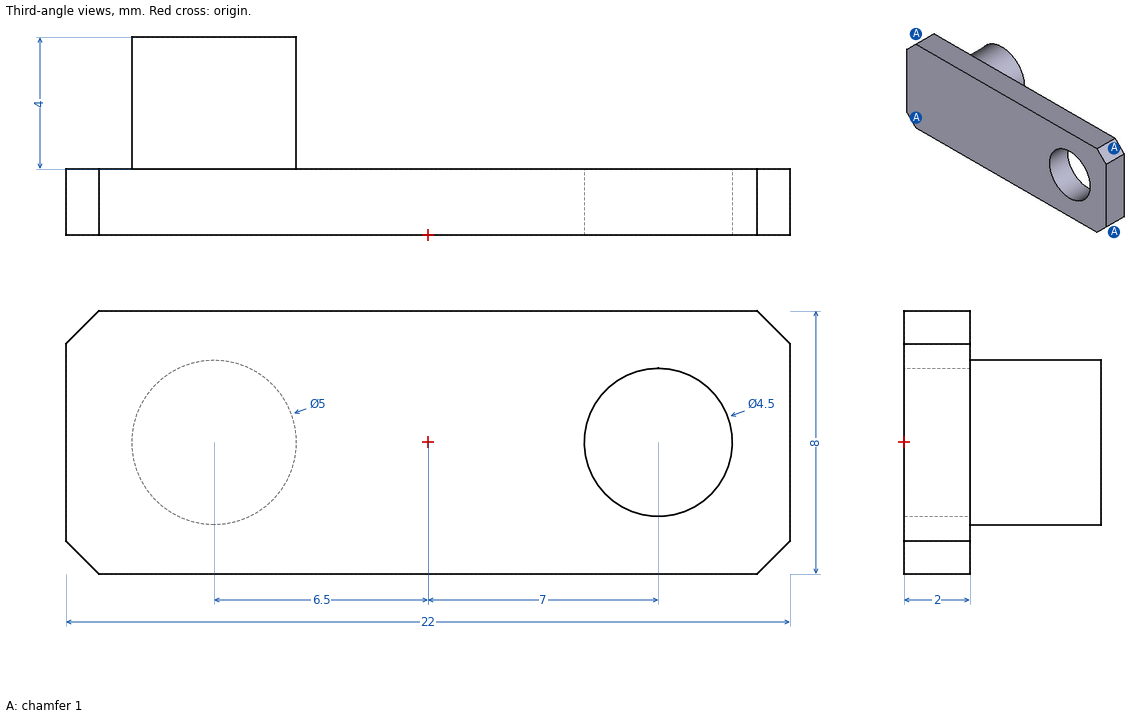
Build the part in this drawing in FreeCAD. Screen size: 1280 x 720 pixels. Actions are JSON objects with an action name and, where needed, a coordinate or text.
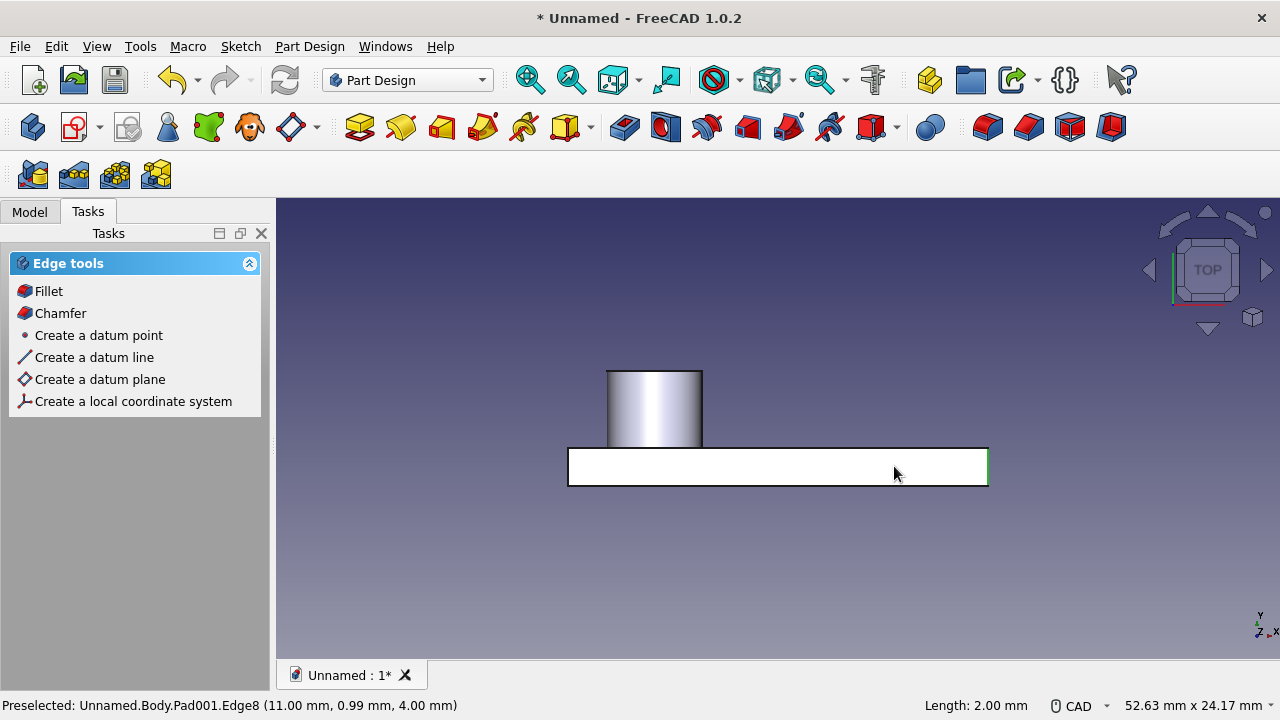
{"action": "left_click", "coordinate": [531, 80]}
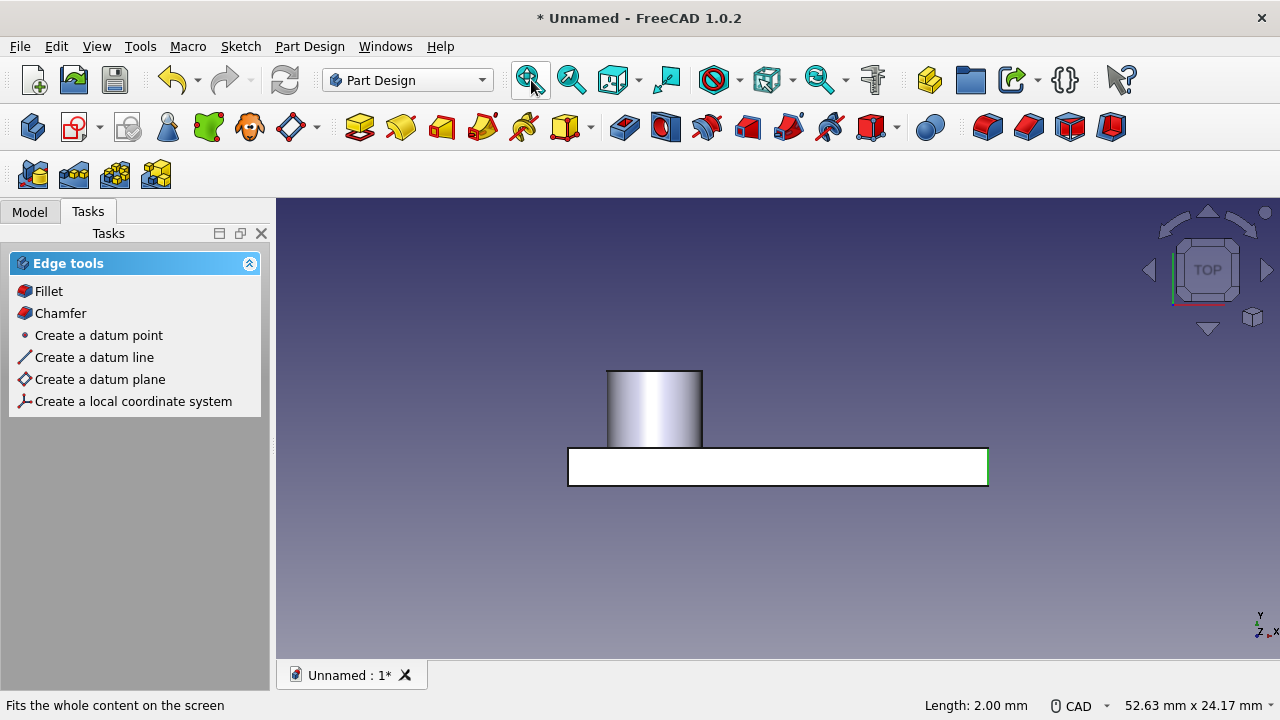
{"action": "left_click", "coordinate": [568, 466], "text": "ctrl"}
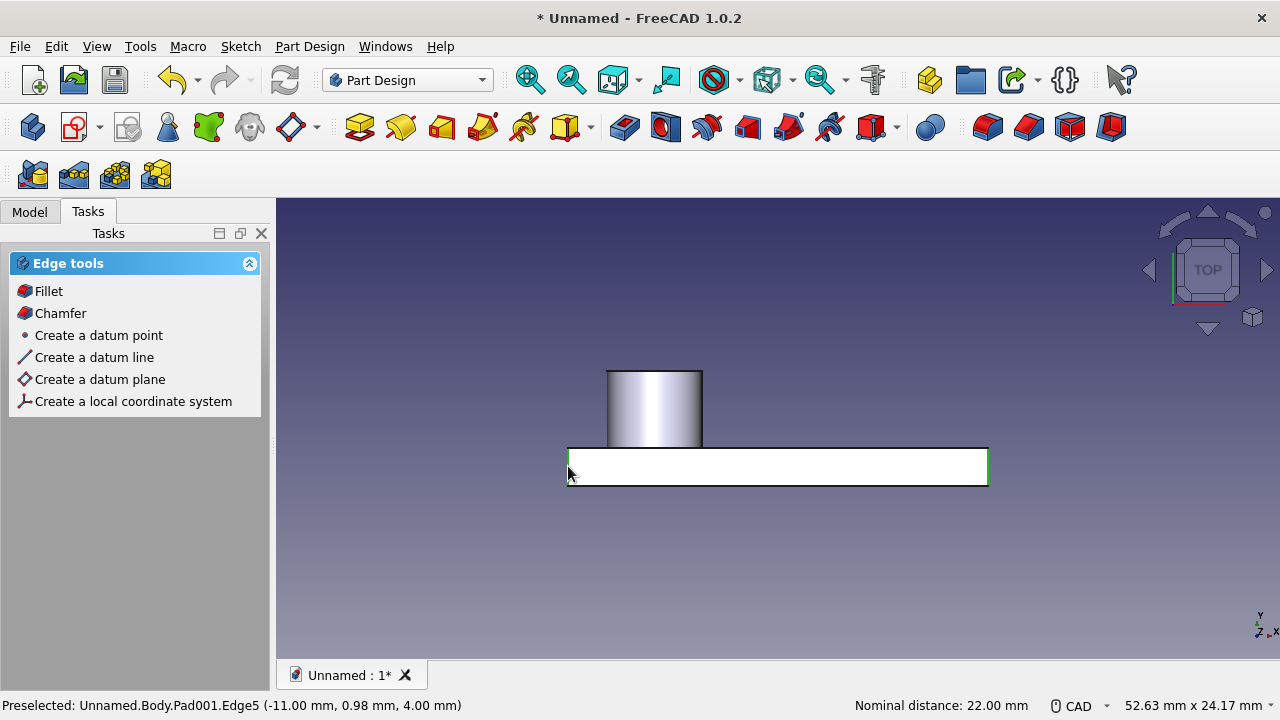
{"action": "key", "text": "1"}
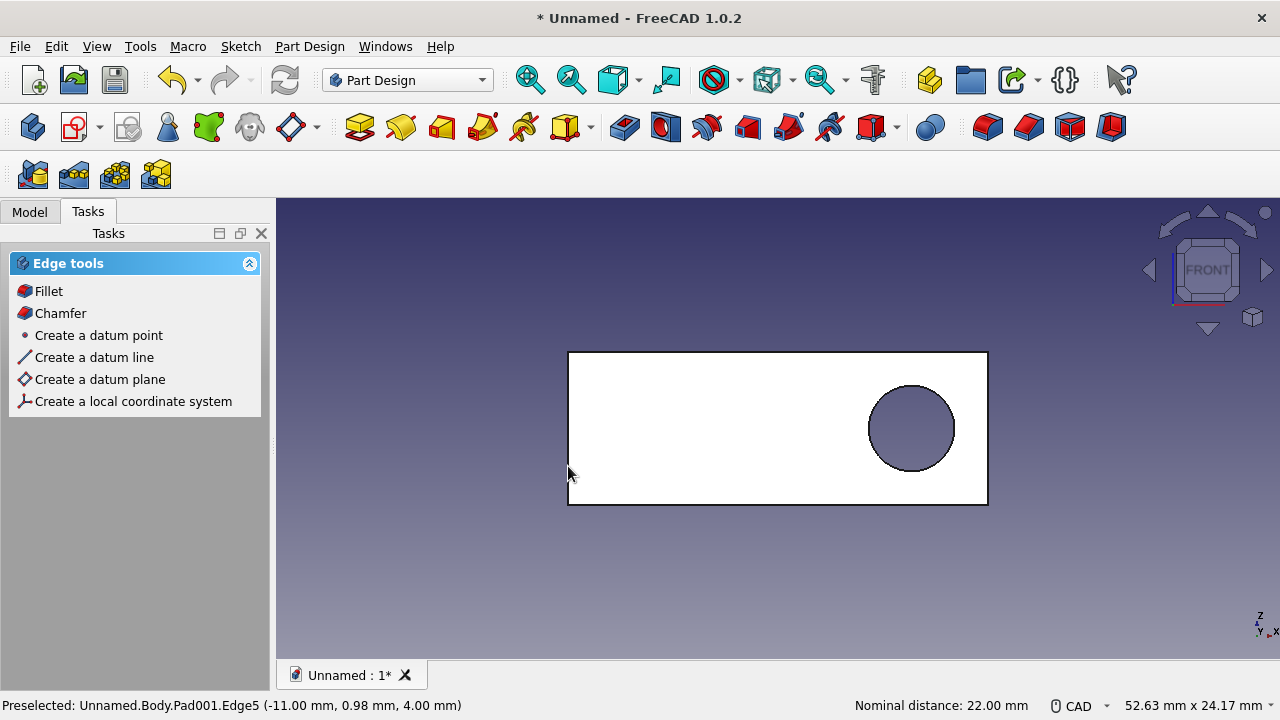
{"action": "key", "text": "v f"}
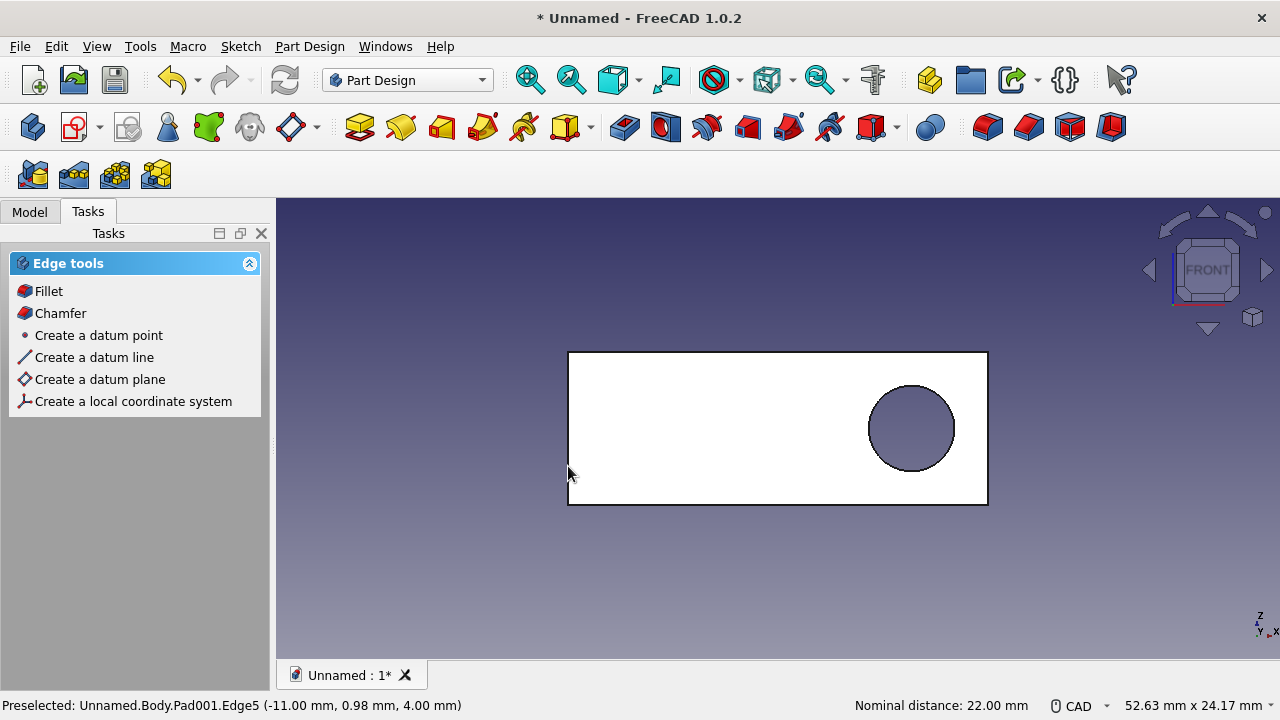
{"action": "key", "text": "3"}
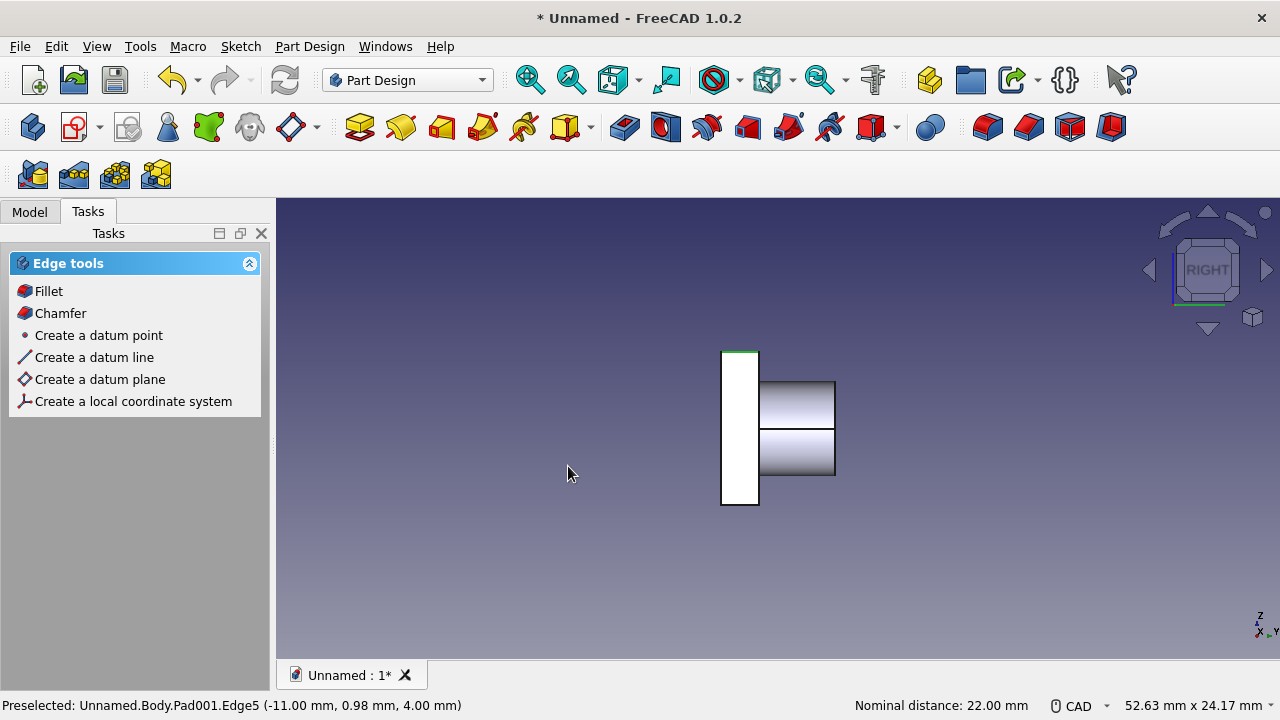
{"action": "left_click", "coordinate": [531, 80]}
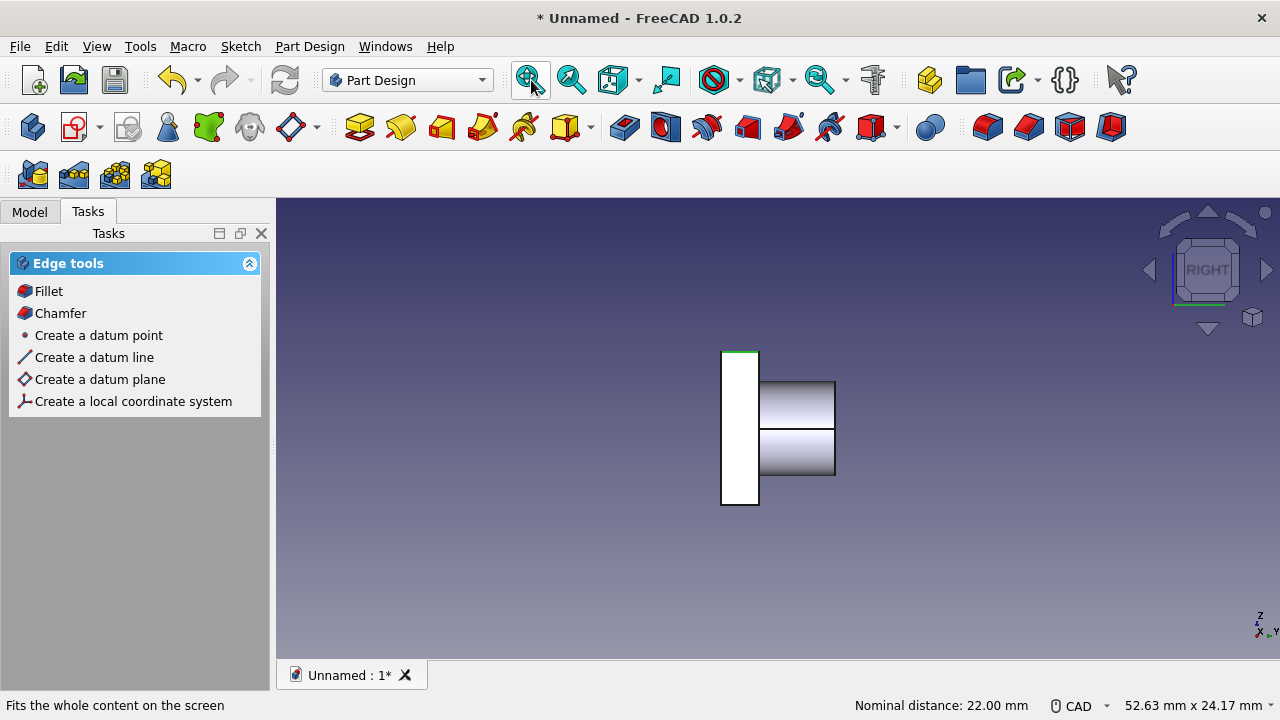
{"action": "left_click", "coordinate": [740, 504], "text": "ctrl"}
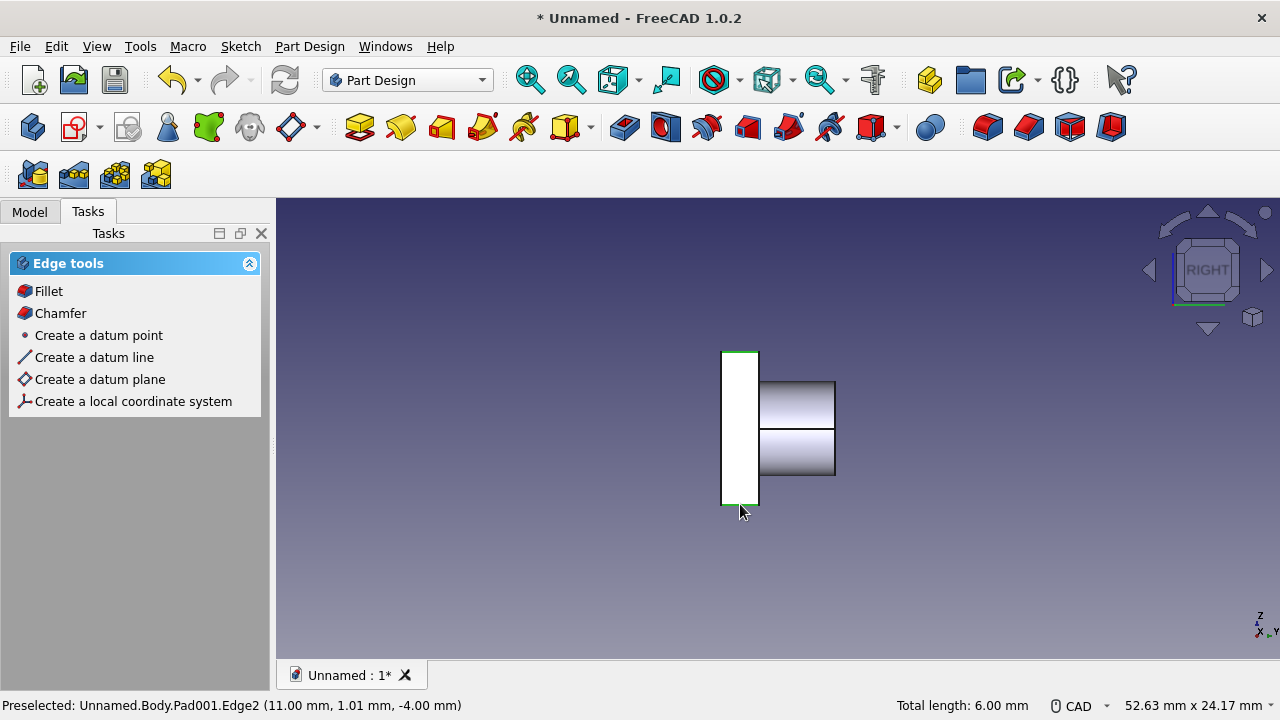
{"action": "key", "text": "5"}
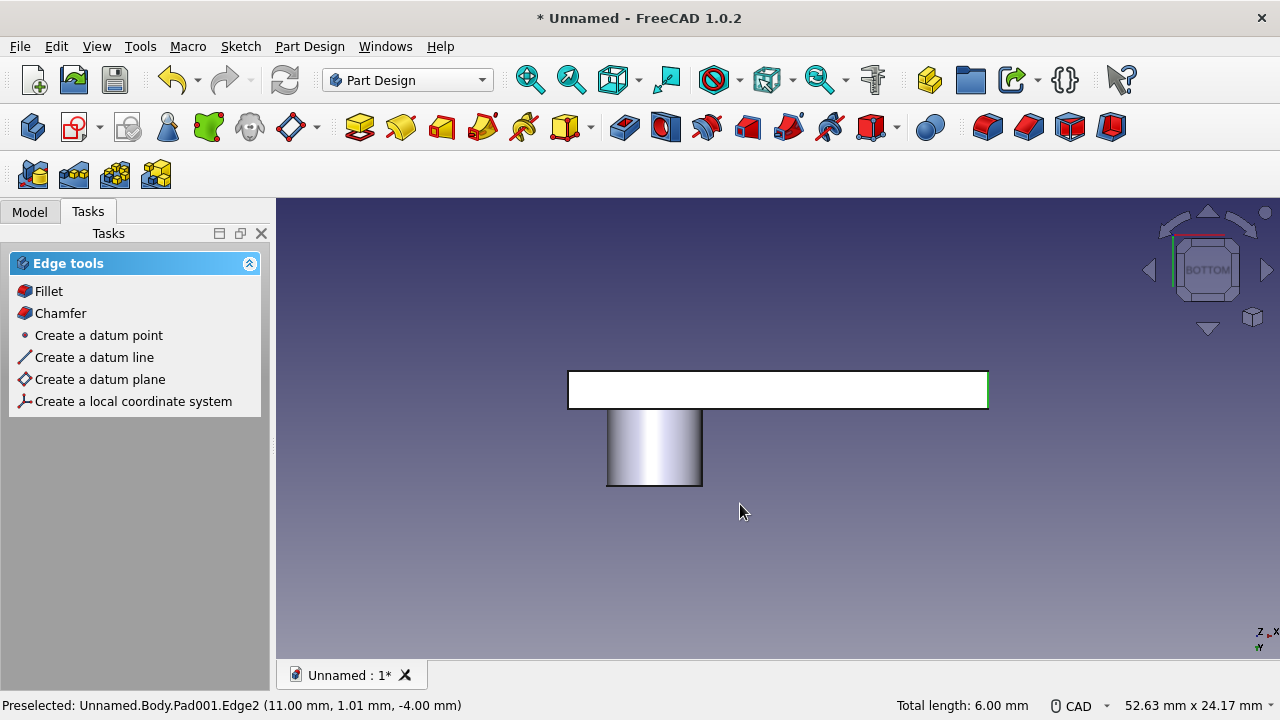
{"action": "left_click", "coordinate": [531, 80]}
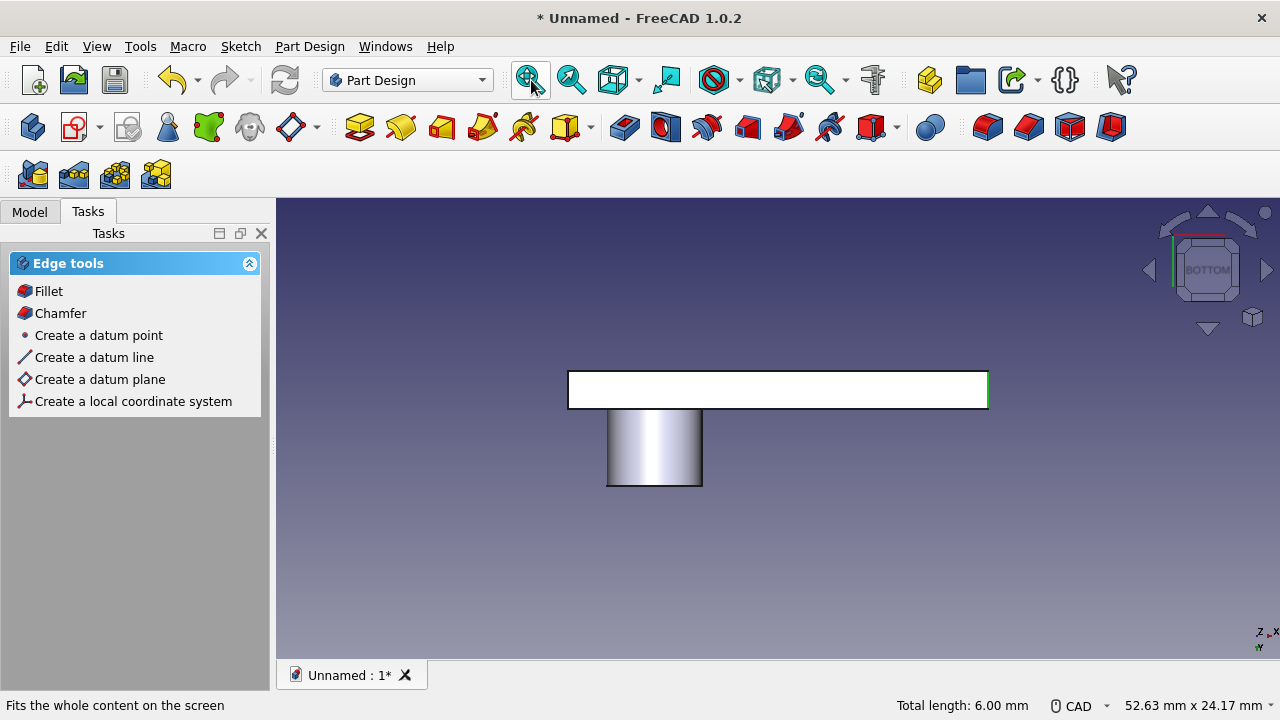
{"action": "left_click", "coordinate": [568, 389], "text": "ctrl"}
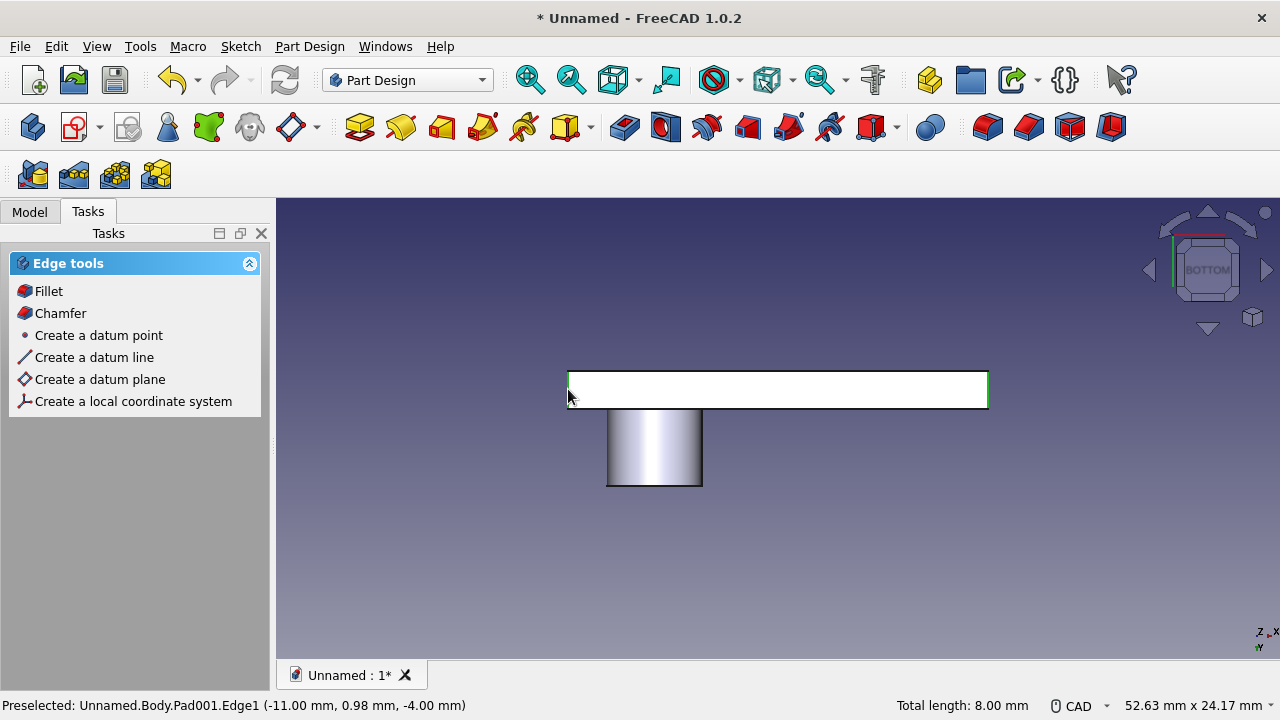
{"action": "left_click", "coordinate": [1029, 128]}